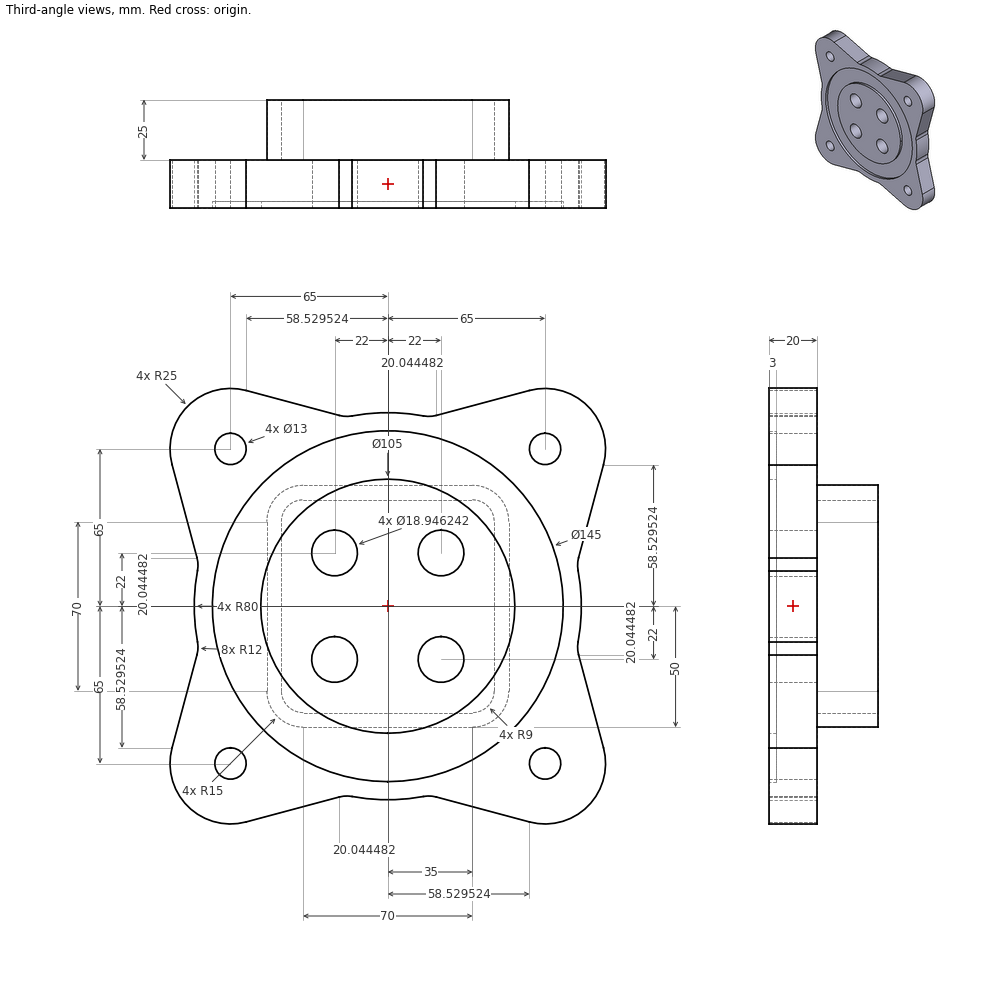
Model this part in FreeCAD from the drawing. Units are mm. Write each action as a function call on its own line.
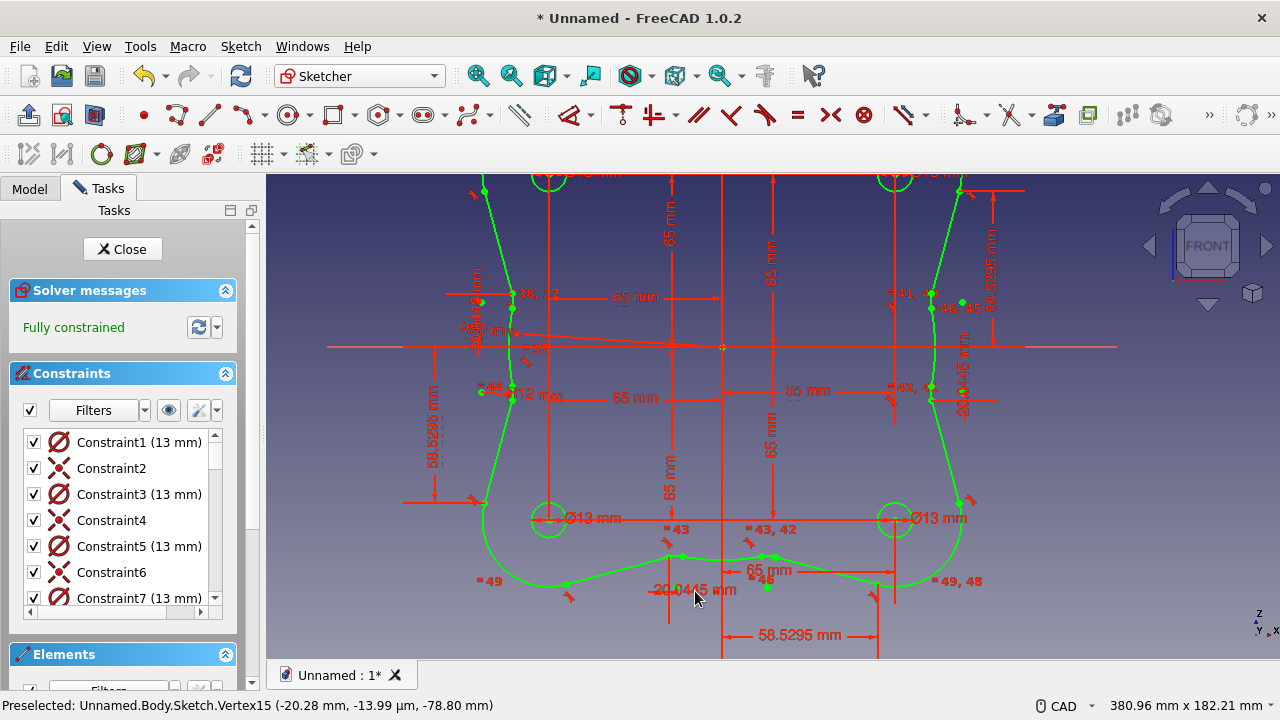
click(123, 249)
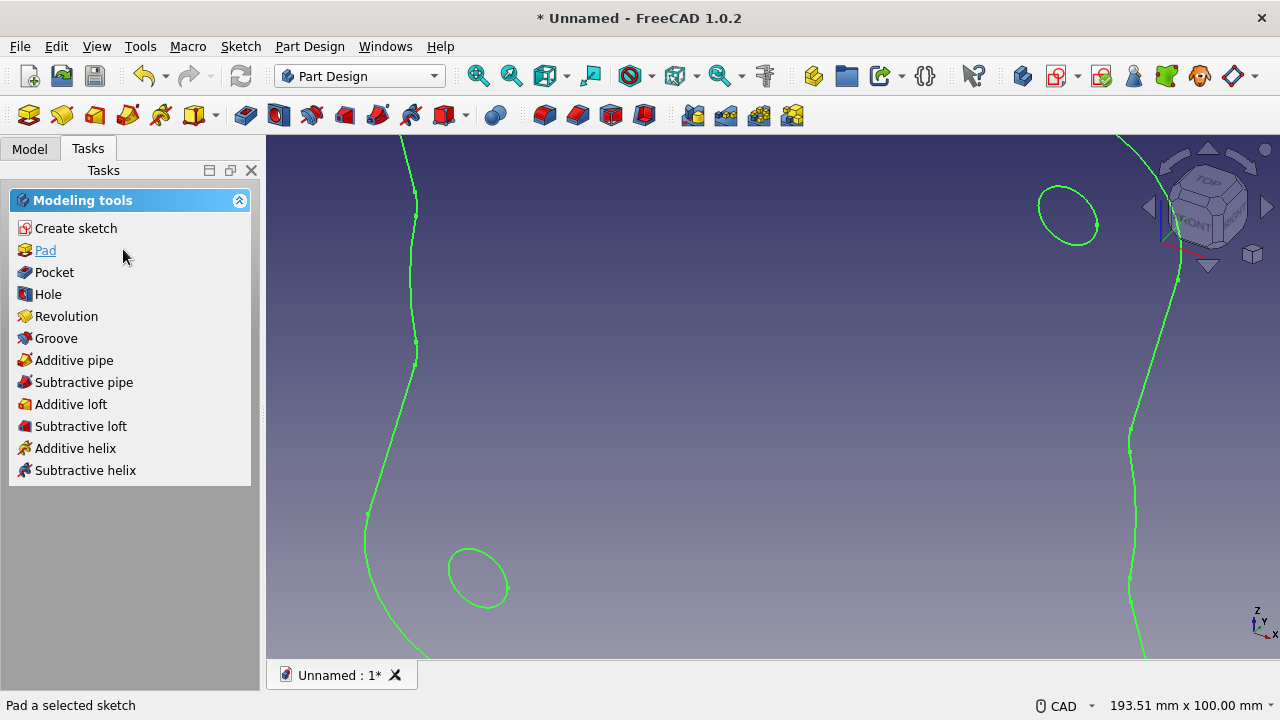
click(29, 116)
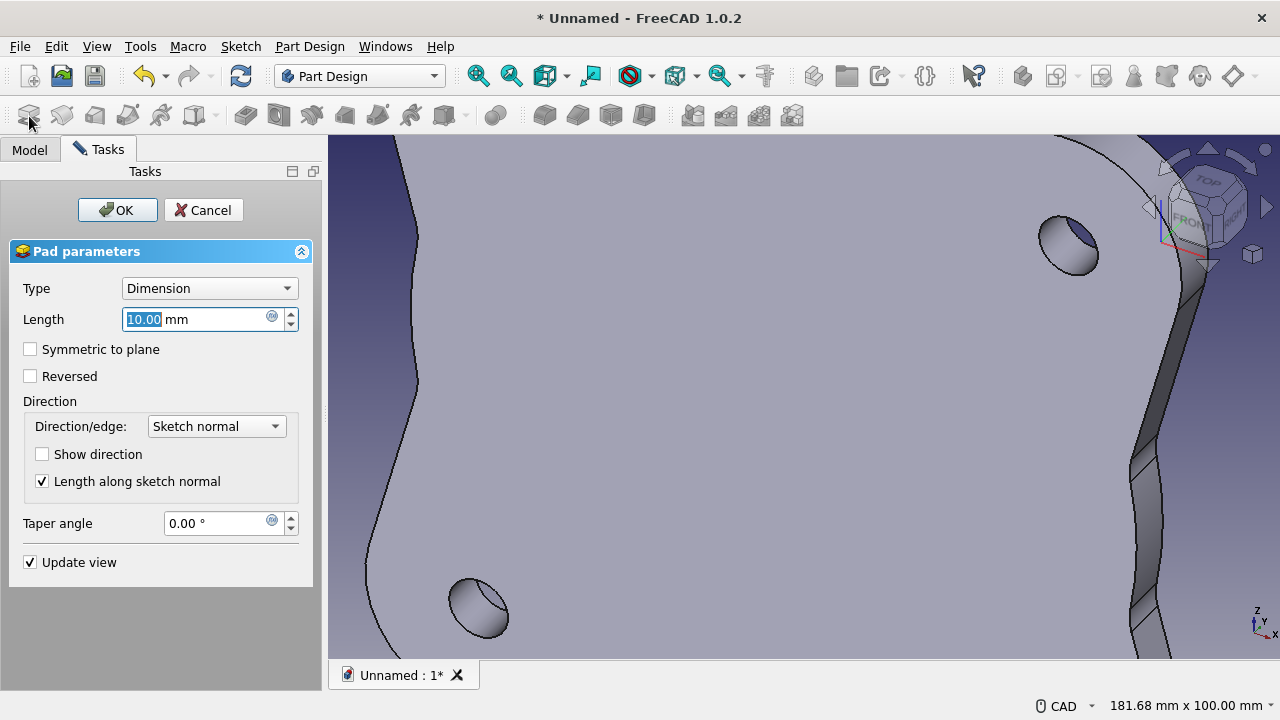
text(20)
key(Tab)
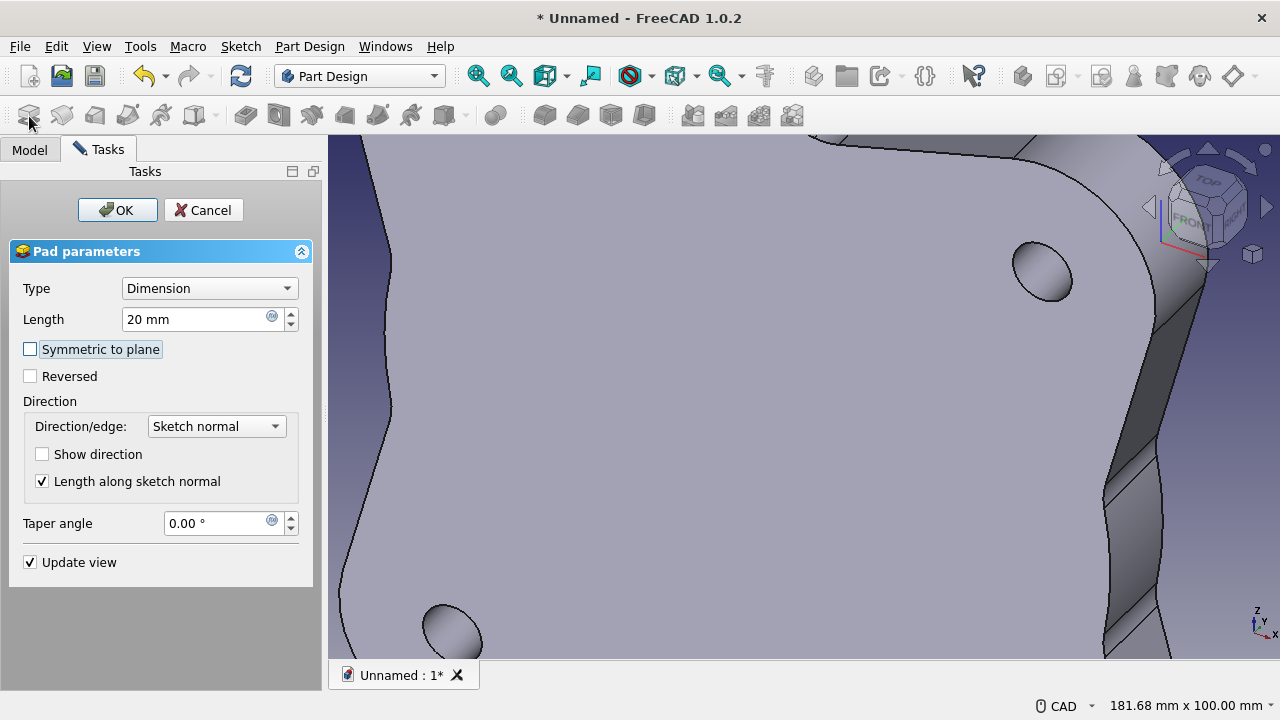
click(31, 349)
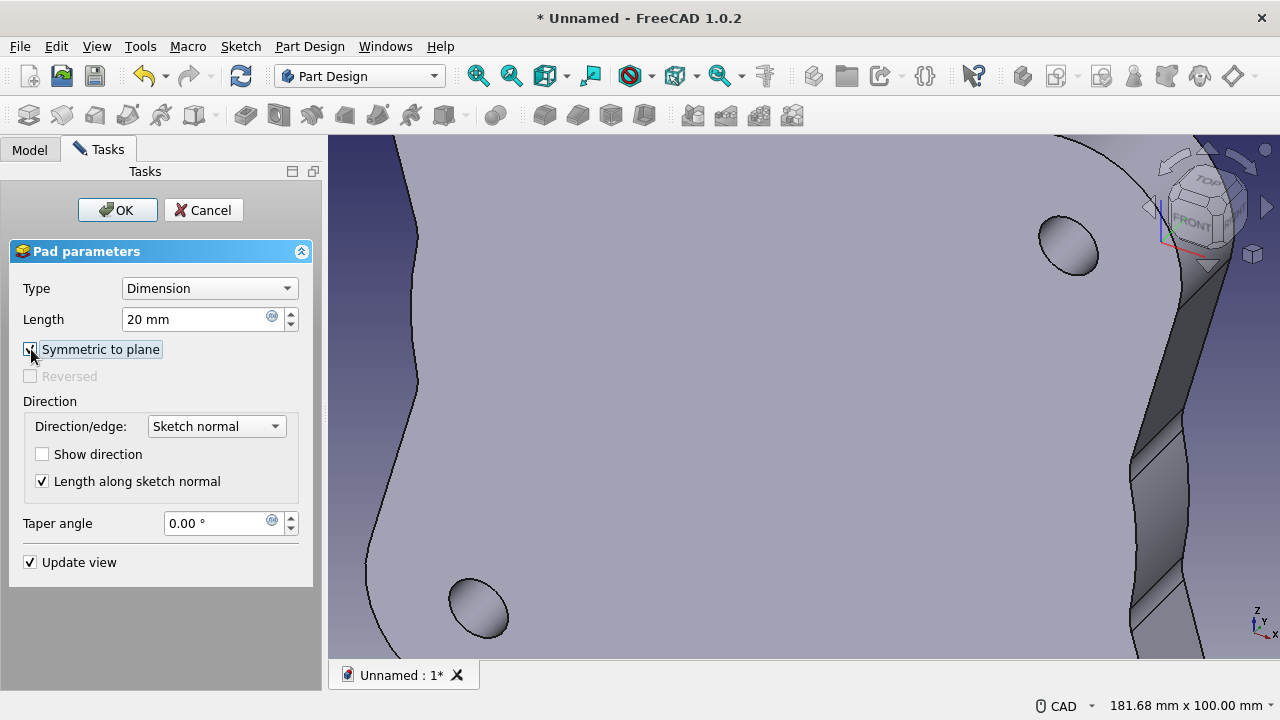
click(118, 210)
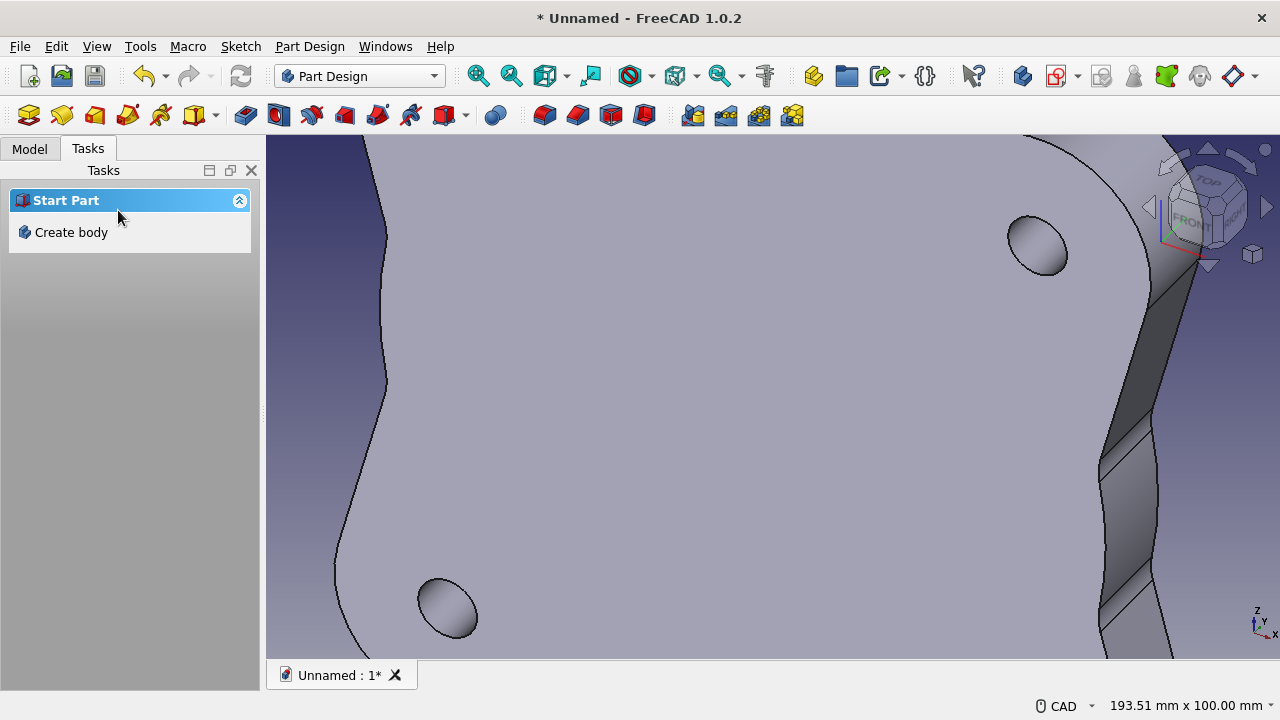
key(v)
key(f)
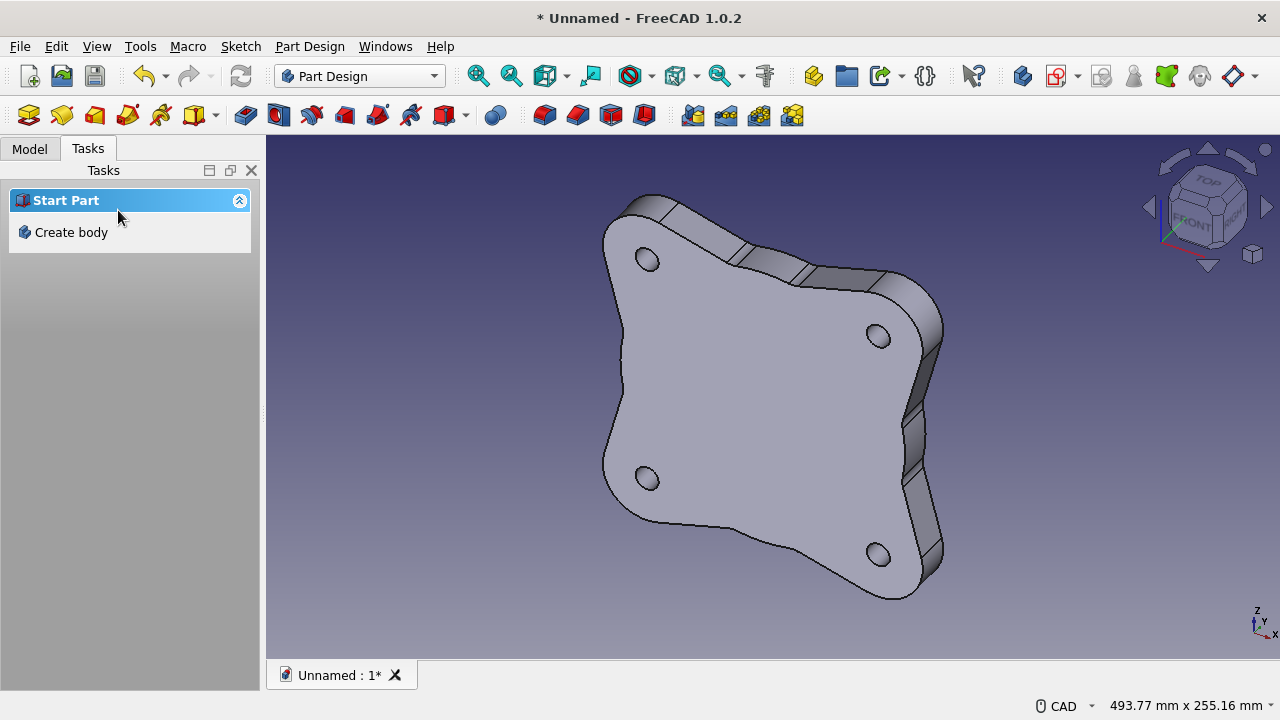
key(4)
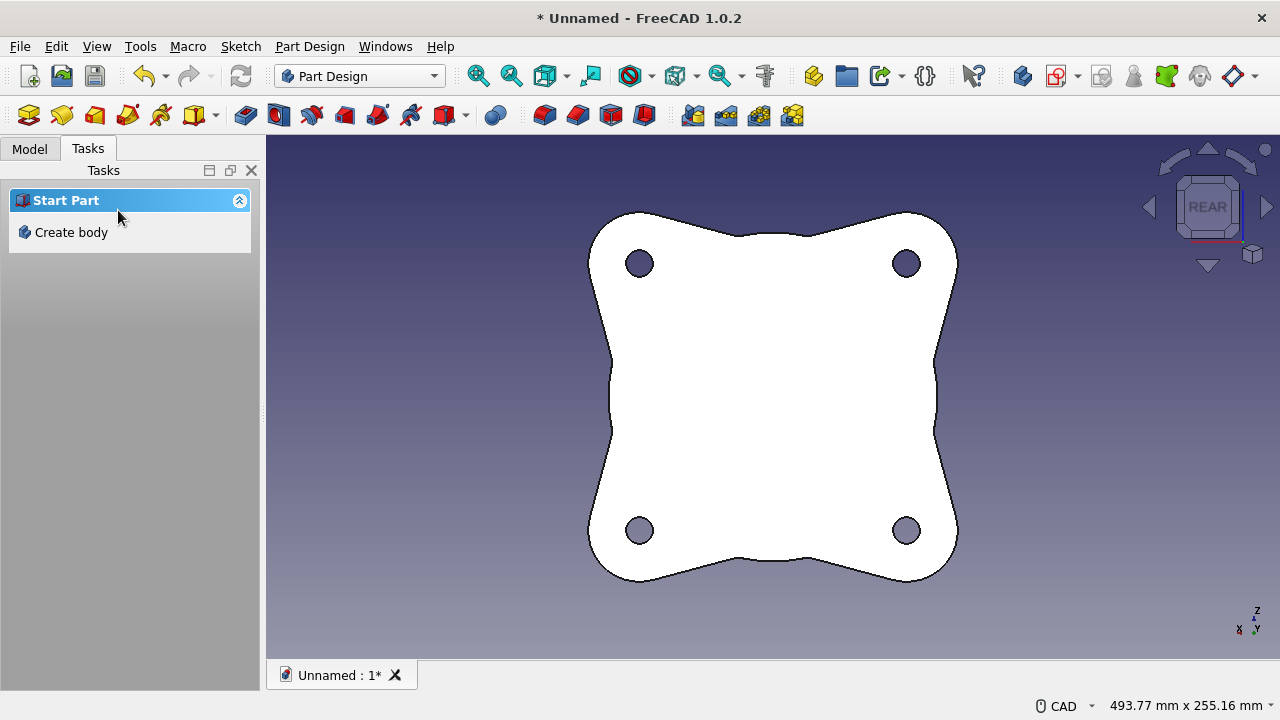
click(773, 396)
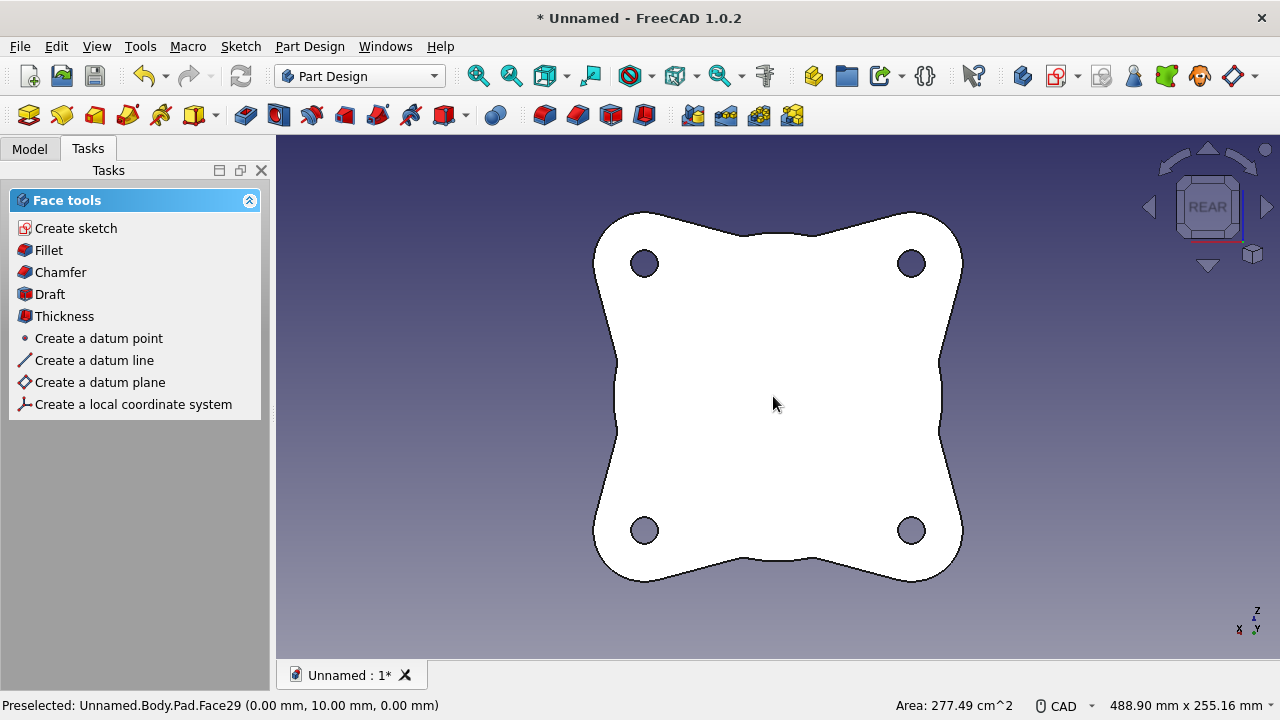
click(1056, 76)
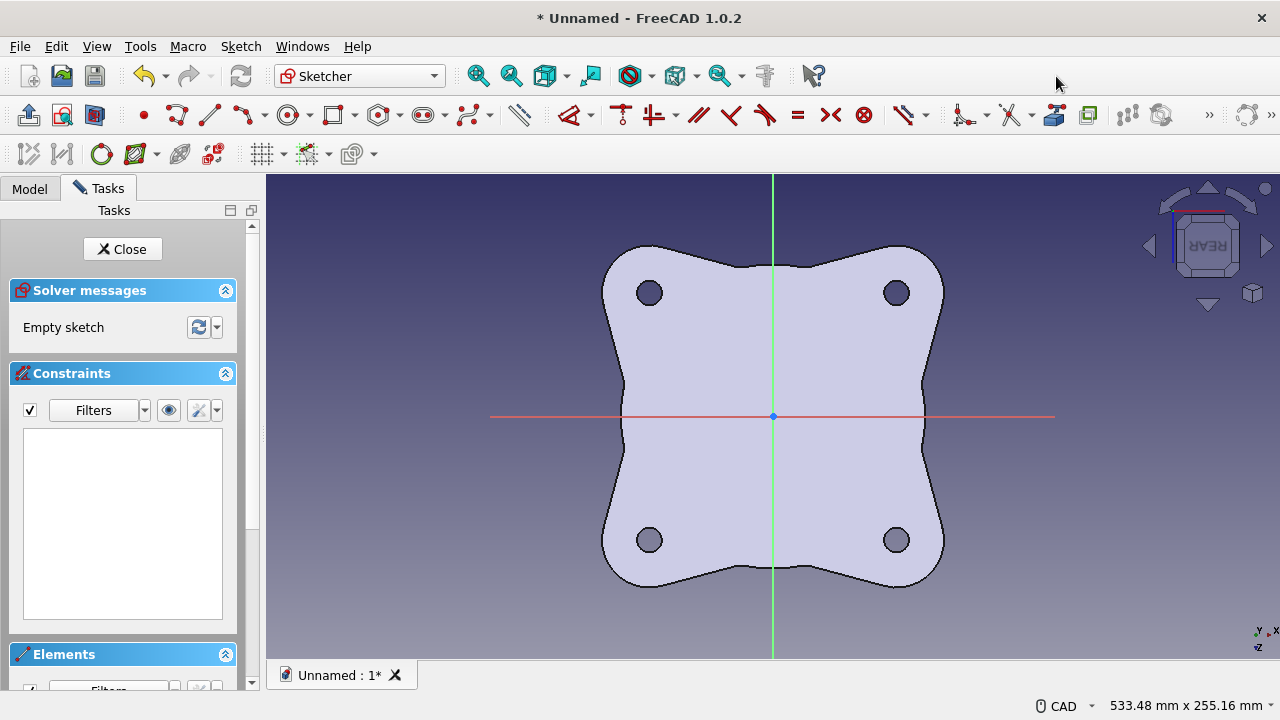
scroll(912, 417, up, 2)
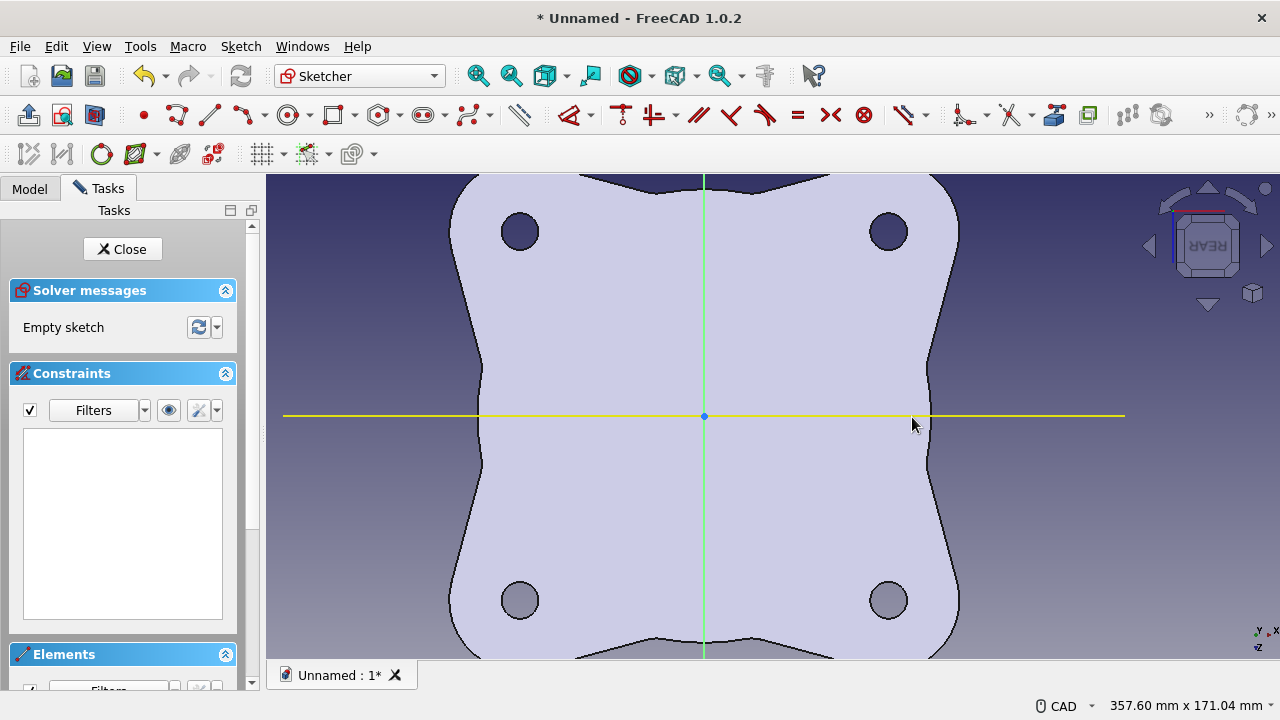
click(210, 116)